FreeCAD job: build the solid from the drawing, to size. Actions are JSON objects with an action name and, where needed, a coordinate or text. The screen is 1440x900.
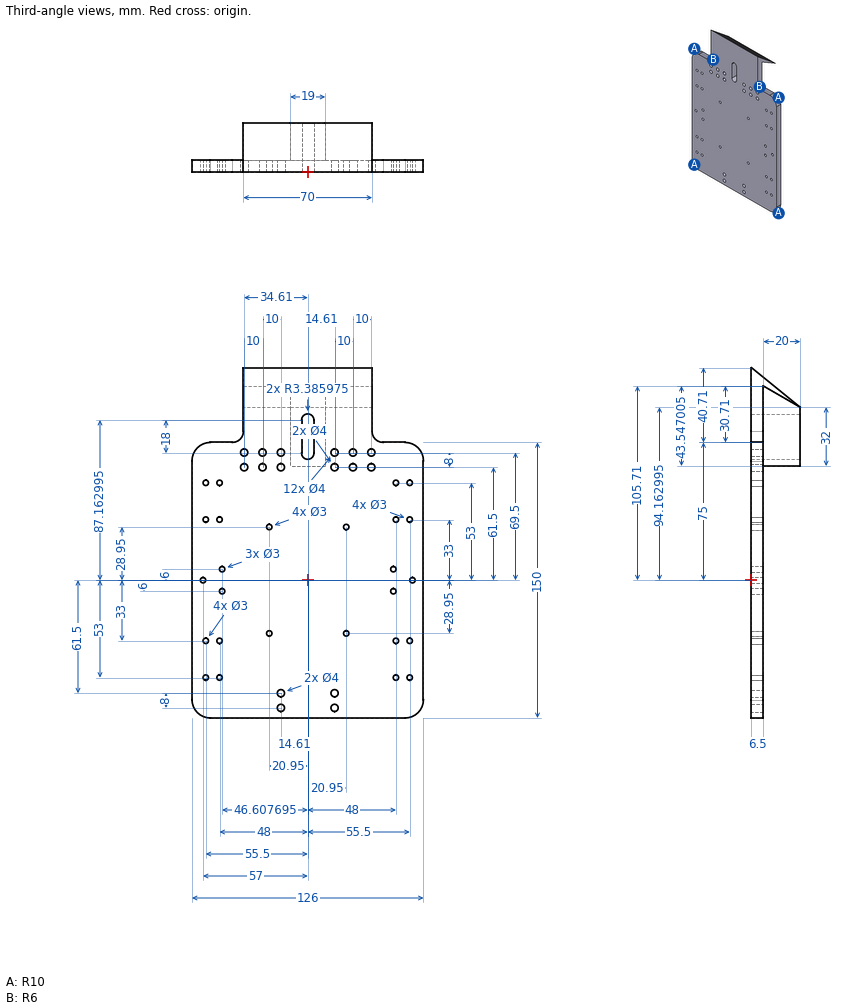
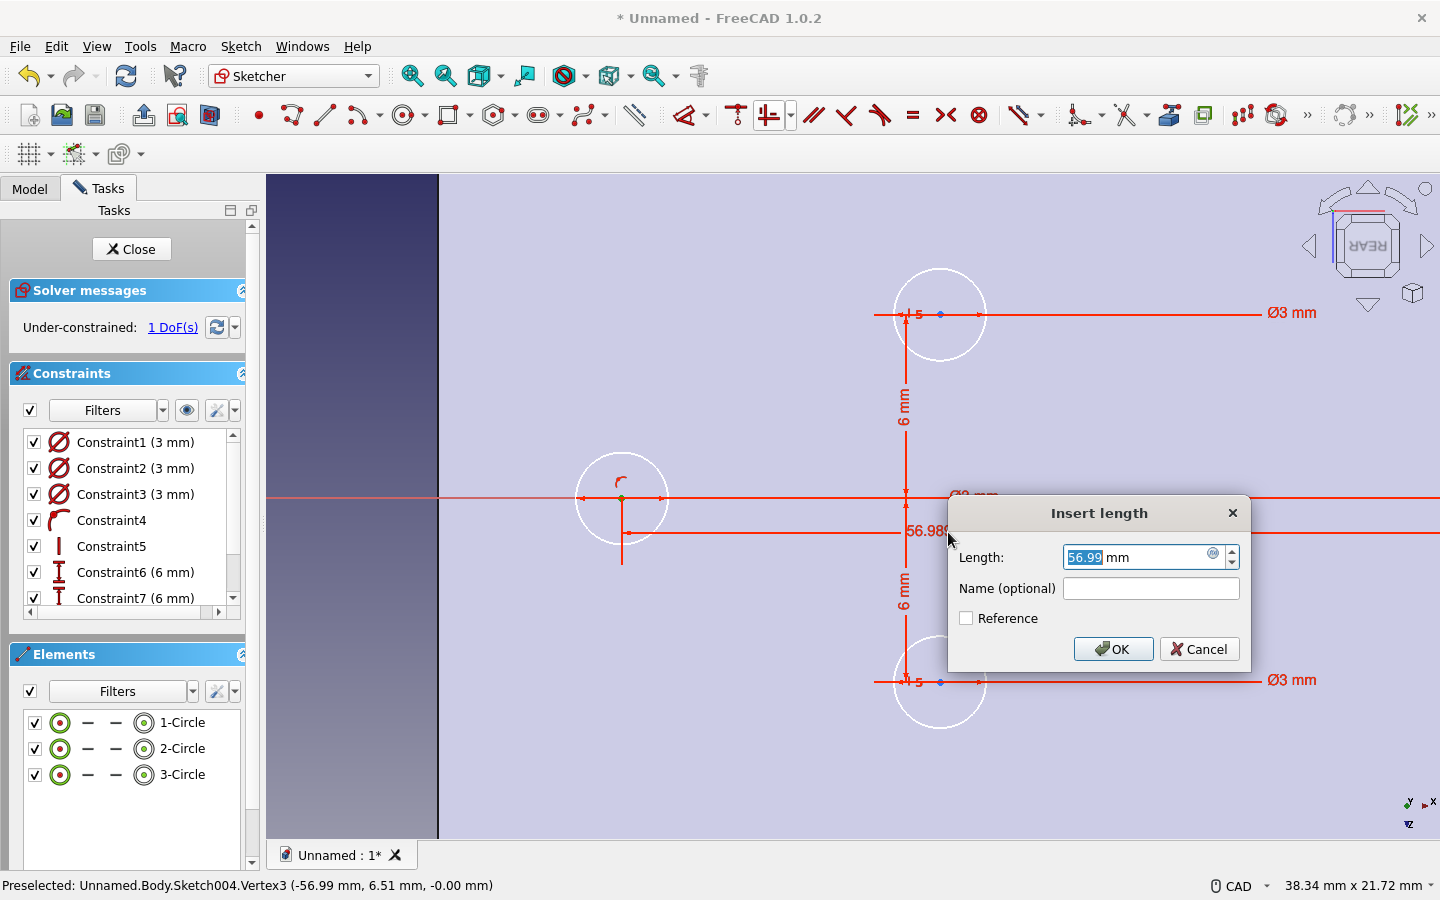
{"action": "type", "text": "57"}
{"action": "key", "text": "Return"}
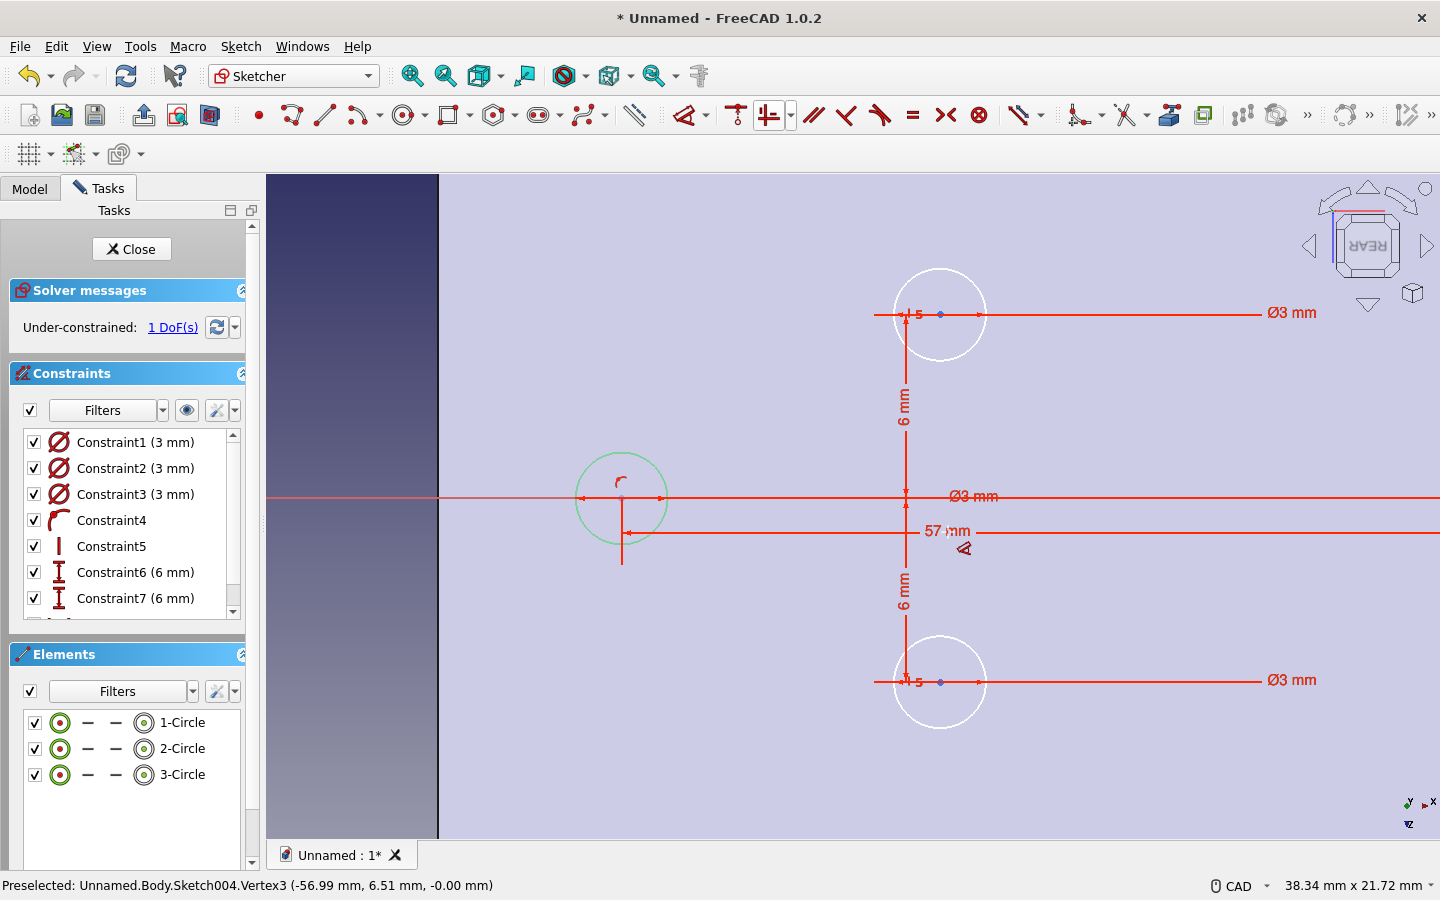
{"action": "left_click", "coordinate": [940, 682]}
{"action": "left_click", "coordinate": [1107, 716]}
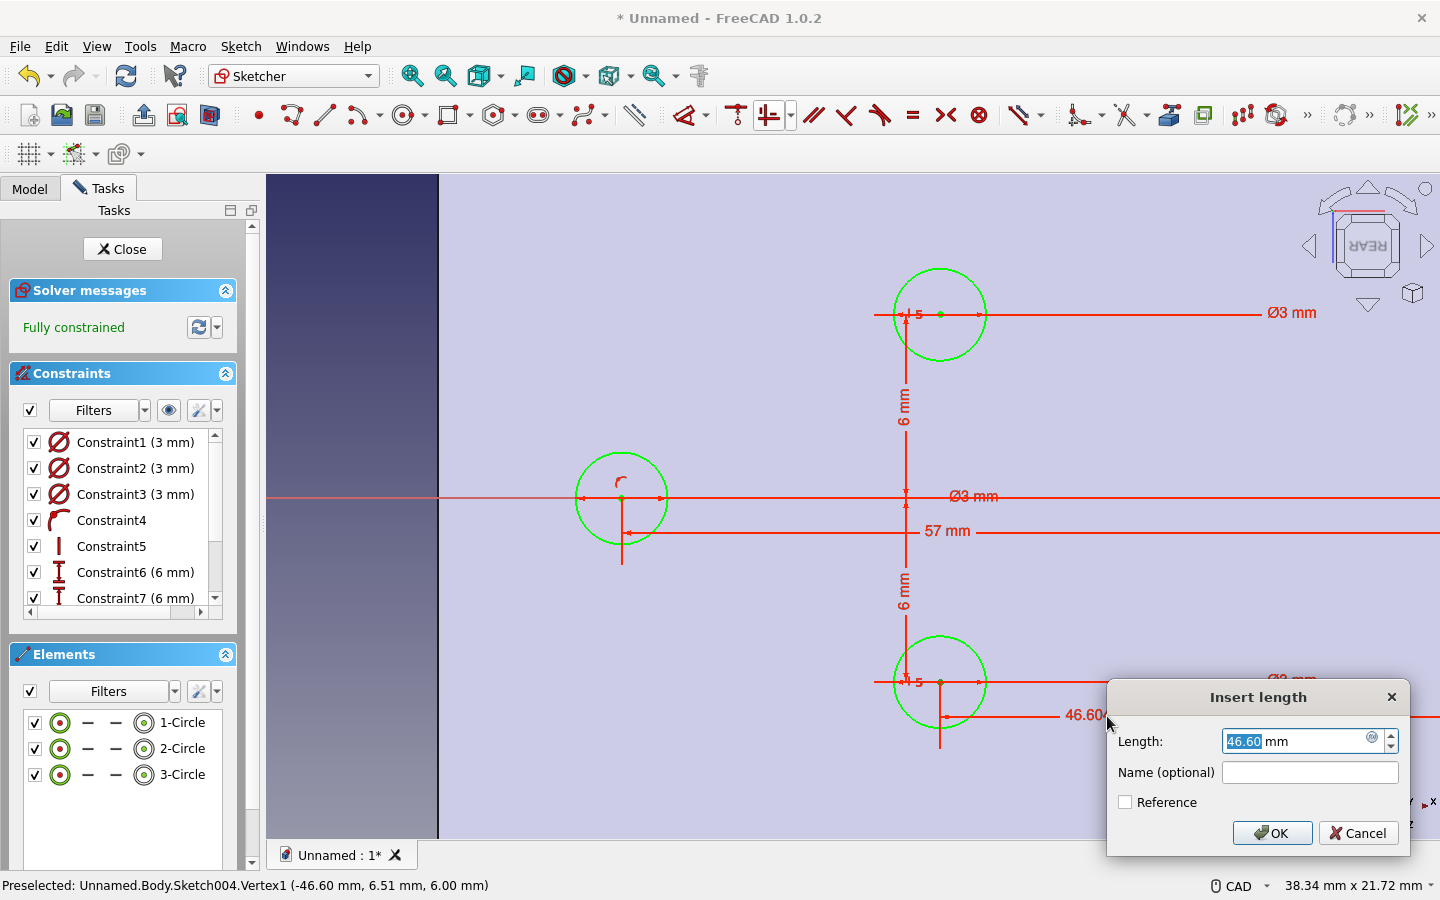
{"action": "type", "text": "46.607695"}
{"action": "key", "text": "Return"}
{"action": "key", "text": "Escape"}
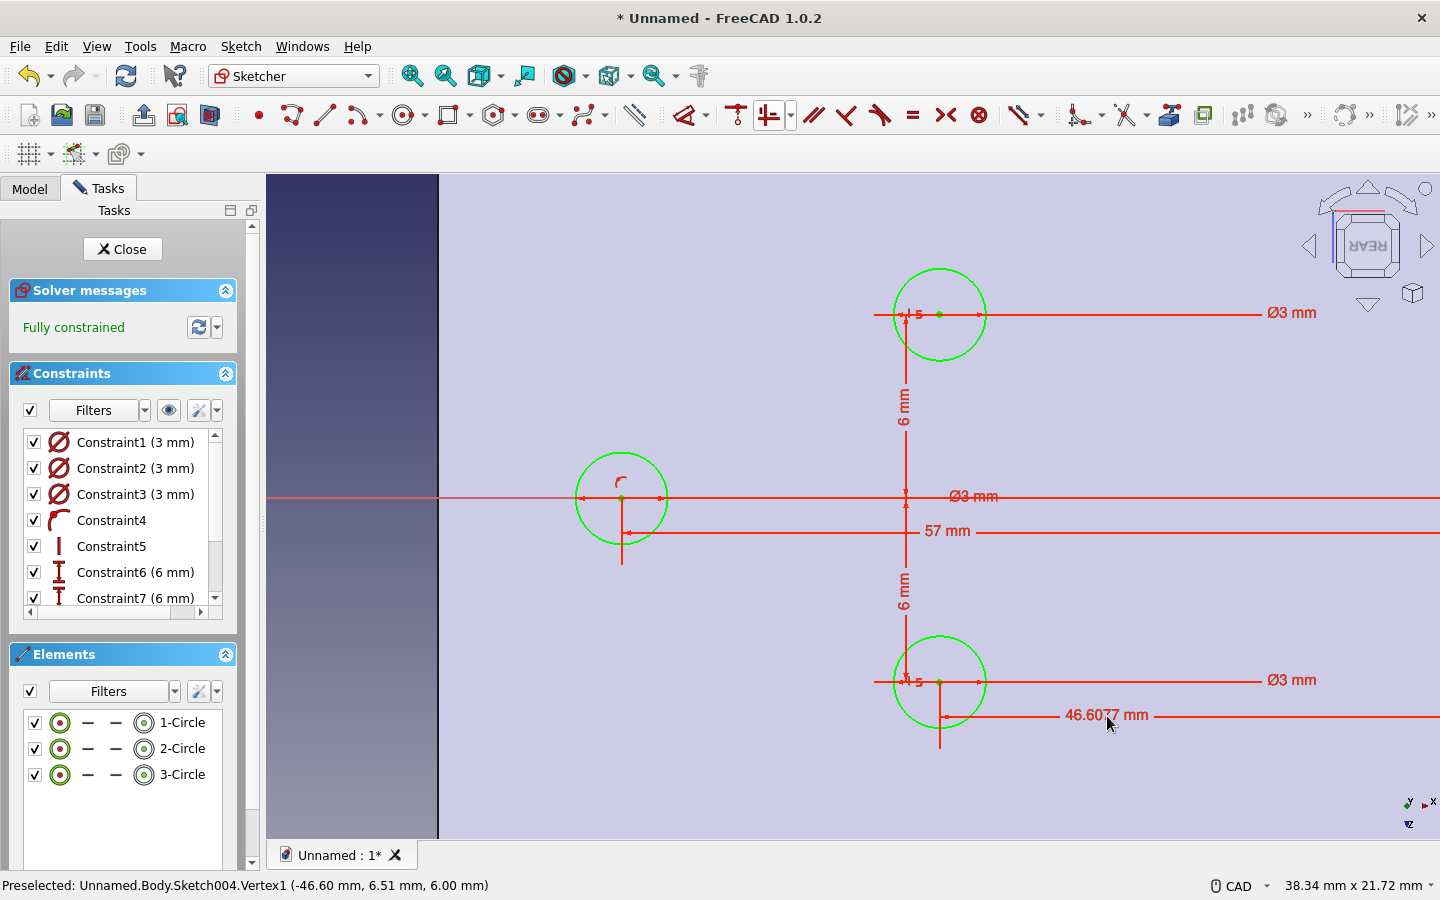
{"action": "left_click", "coordinate": [123, 249]}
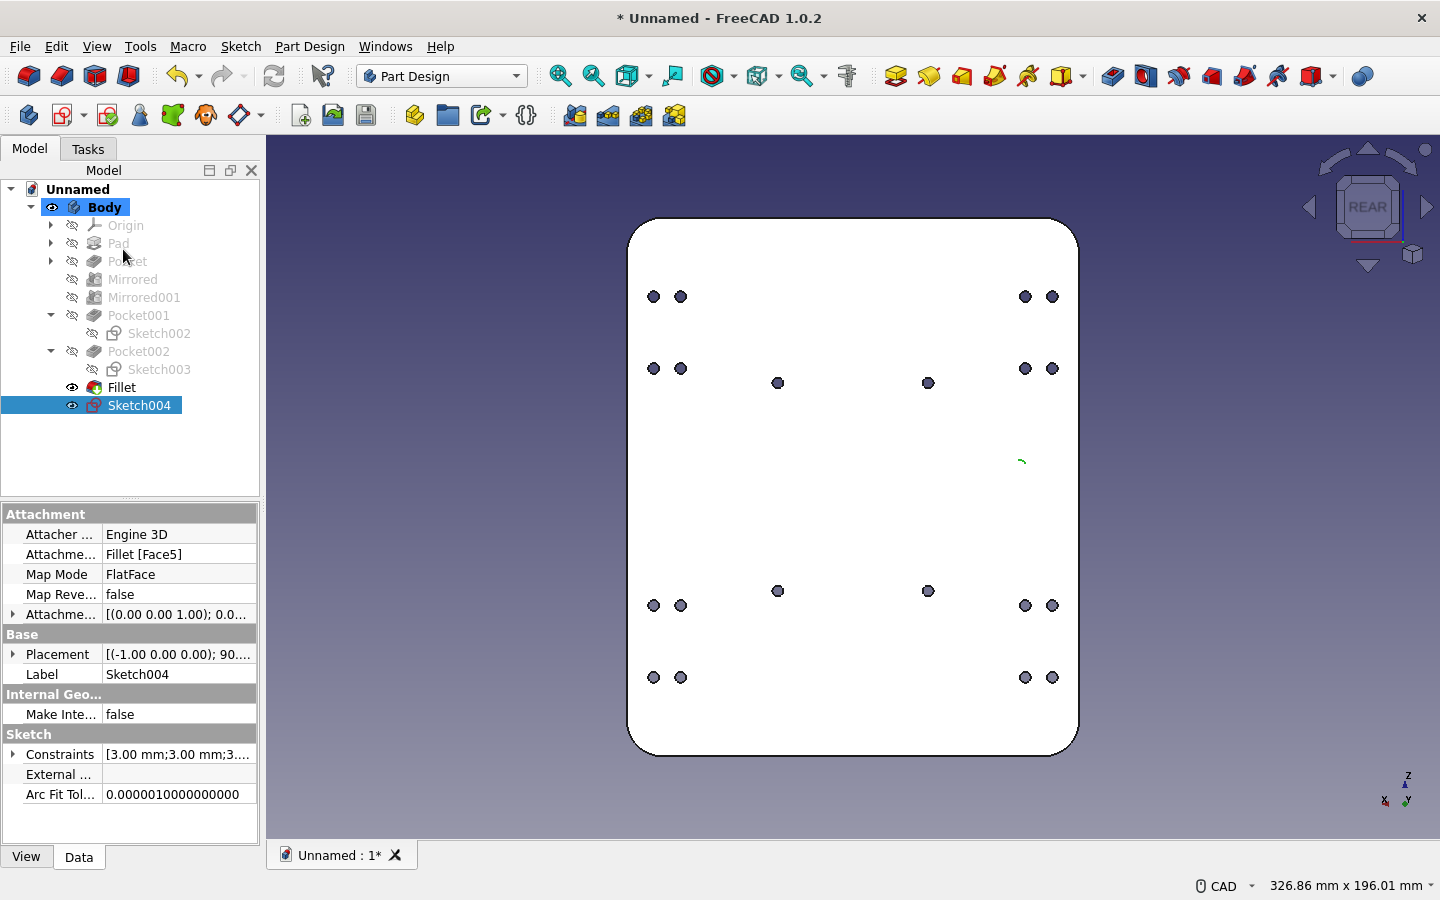
{"action": "left_click", "coordinate": [1113, 76]}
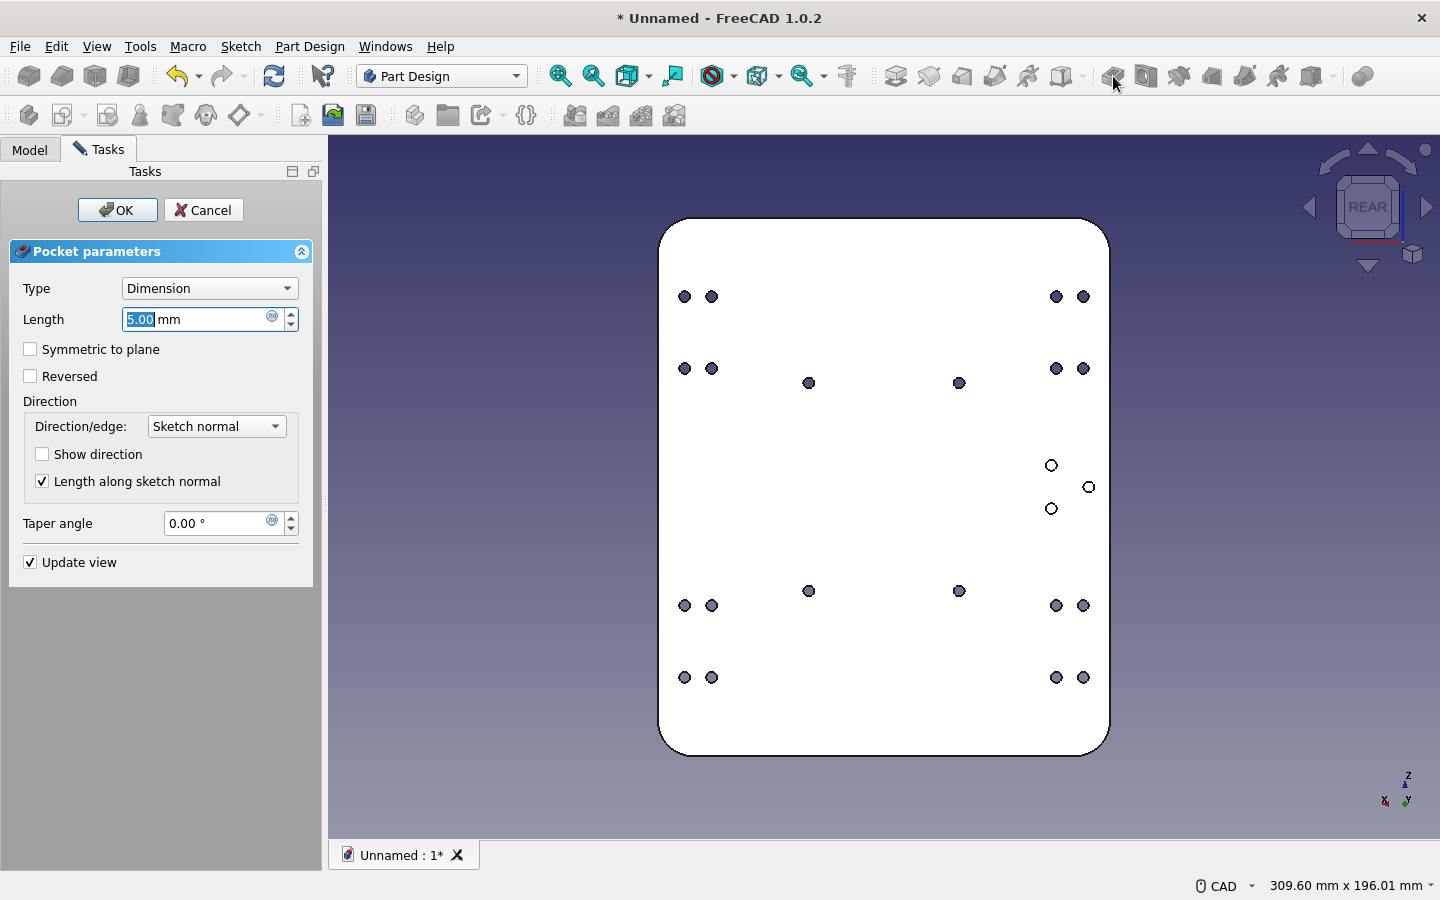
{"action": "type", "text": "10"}
{"action": "key", "text": "Tab"}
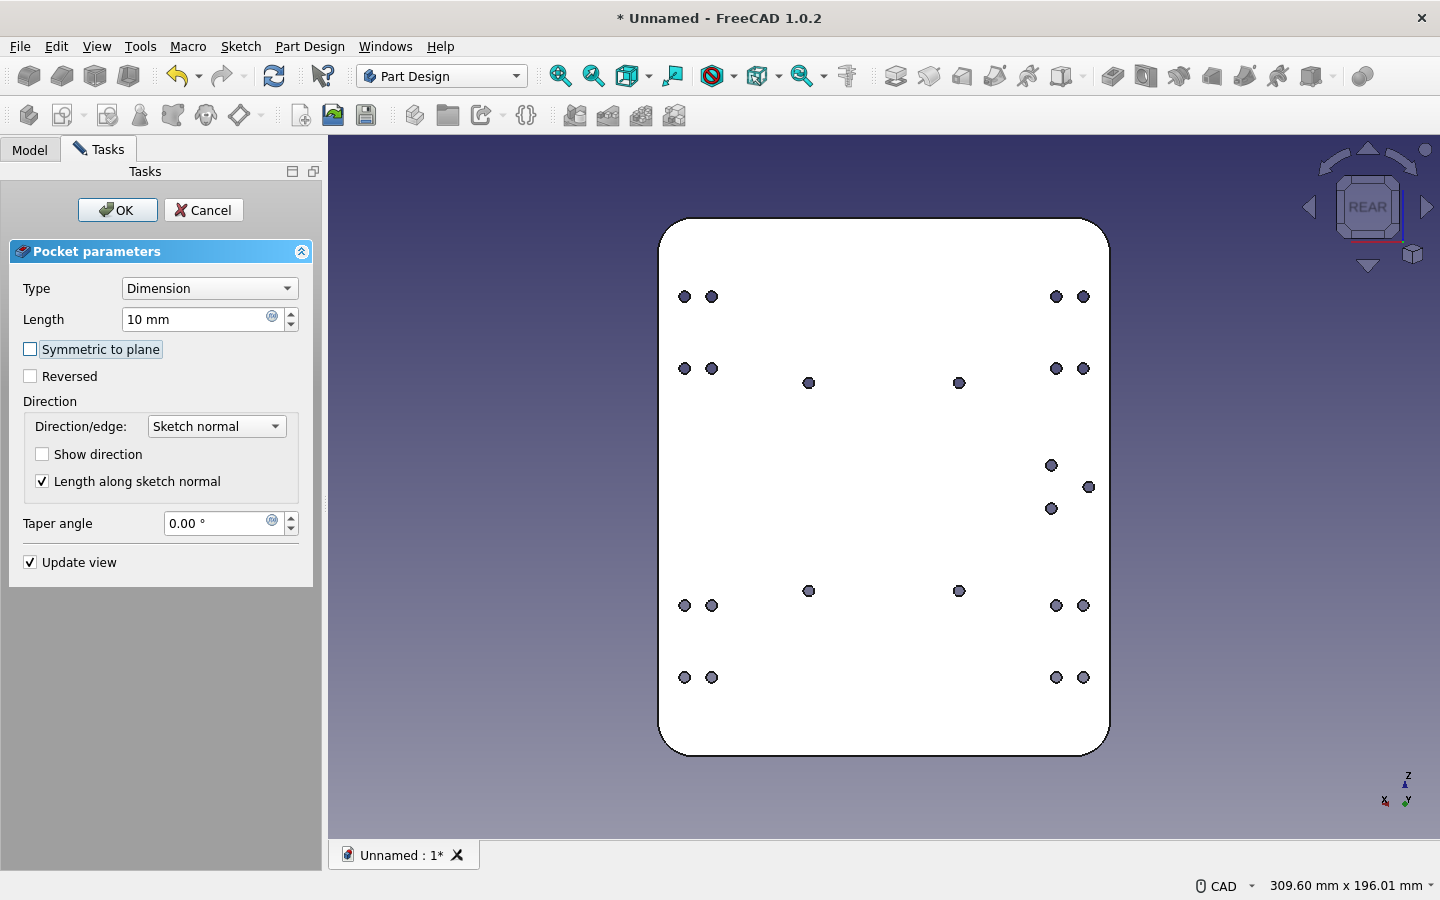
{"action": "left_click", "coordinate": [118, 210]}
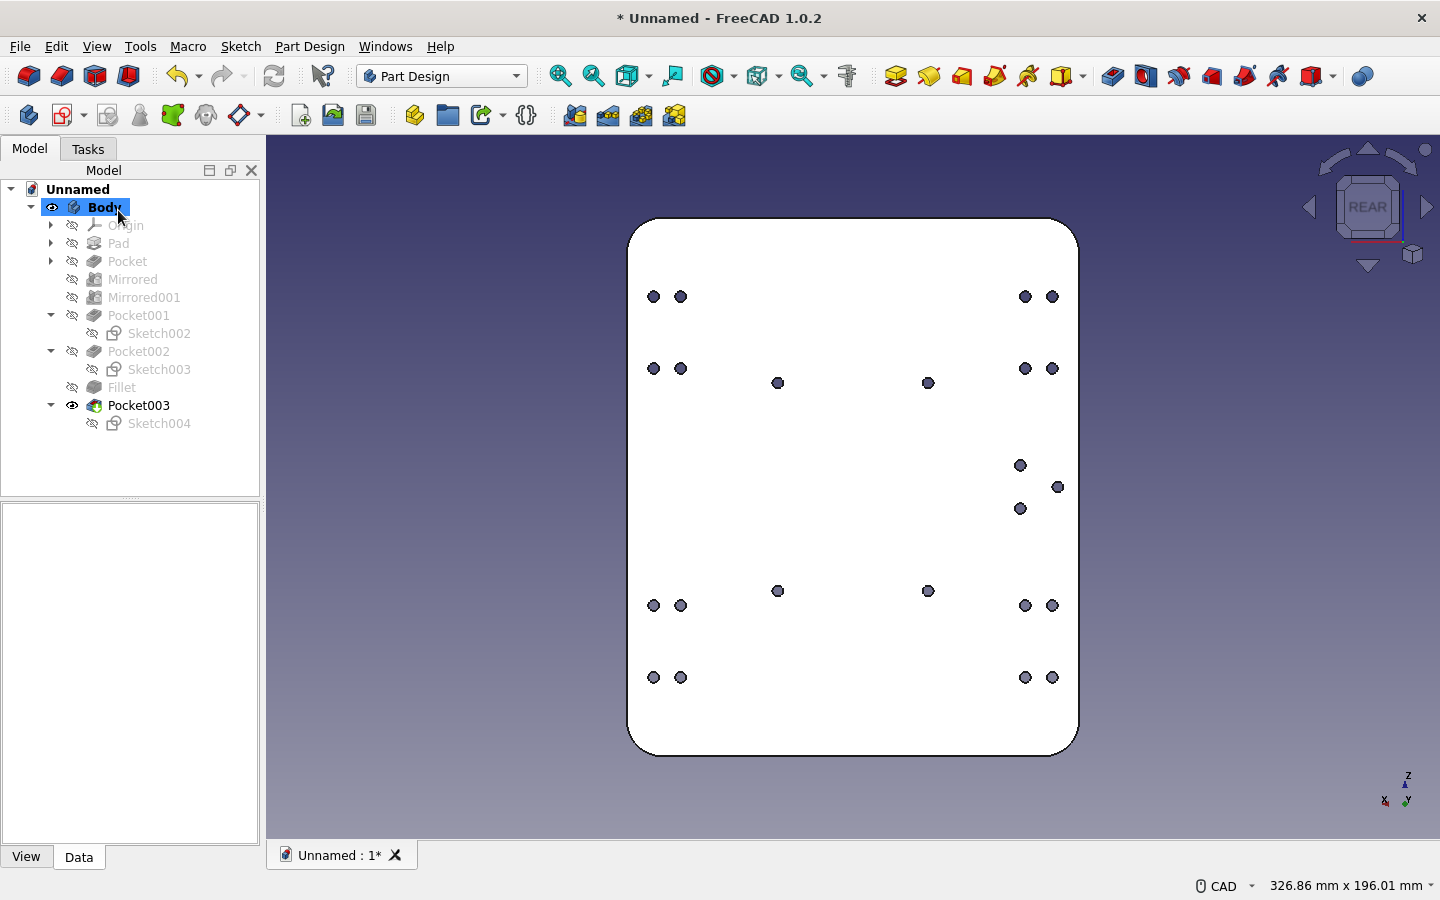
{"action": "left_click", "coordinate": [117, 405]}